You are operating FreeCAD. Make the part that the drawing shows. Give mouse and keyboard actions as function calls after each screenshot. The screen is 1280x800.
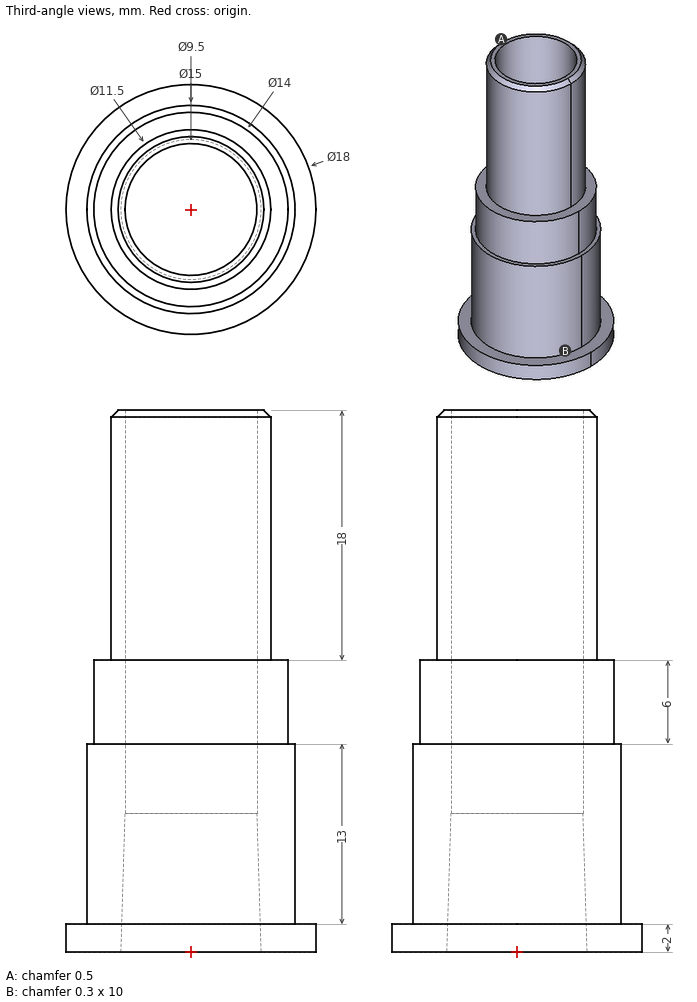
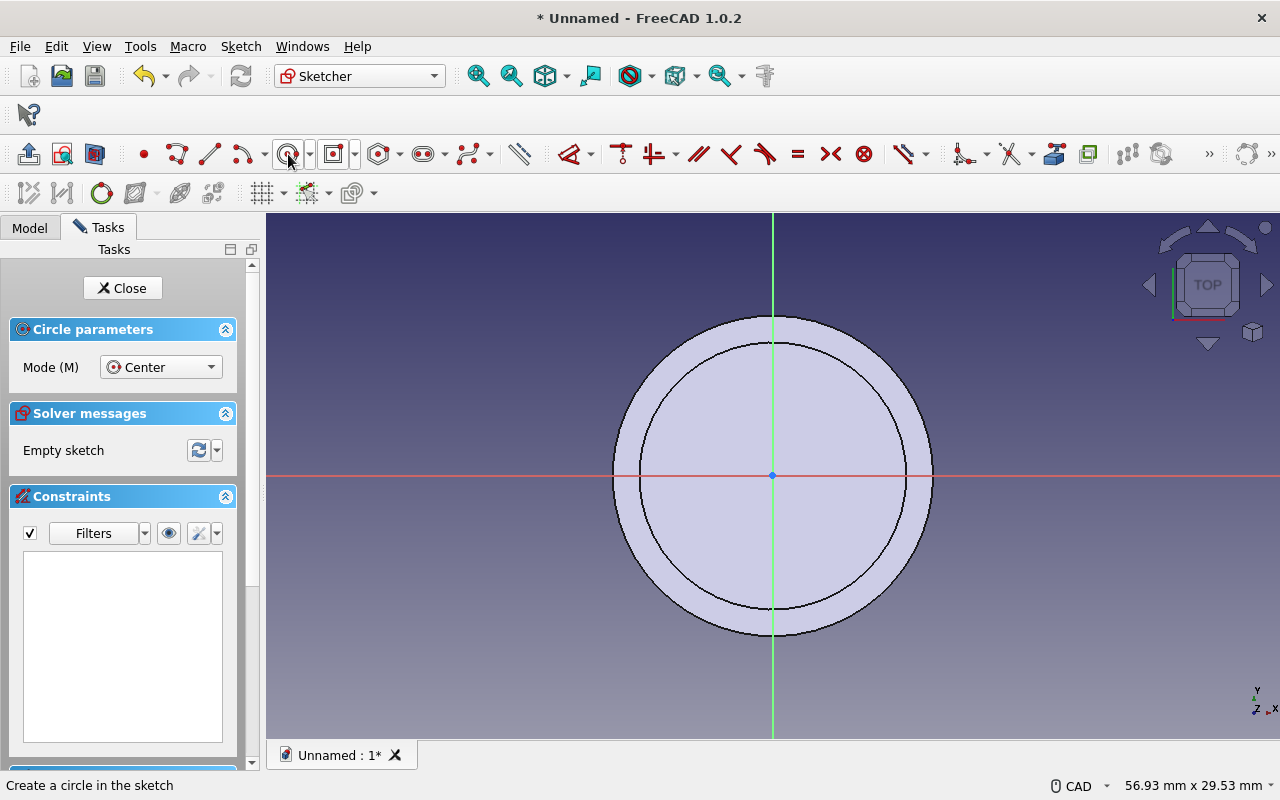
click(773, 476)
click(861, 388)
key(Escape)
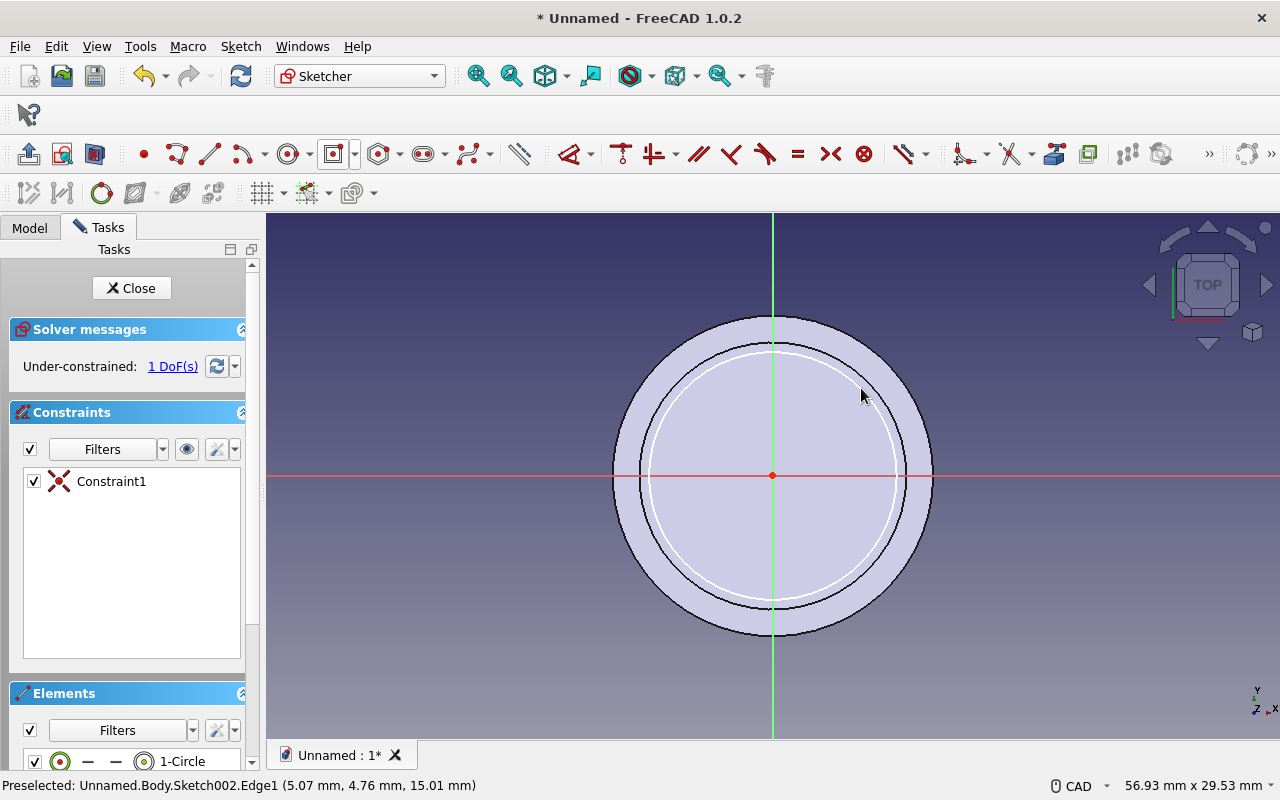
click(568, 154)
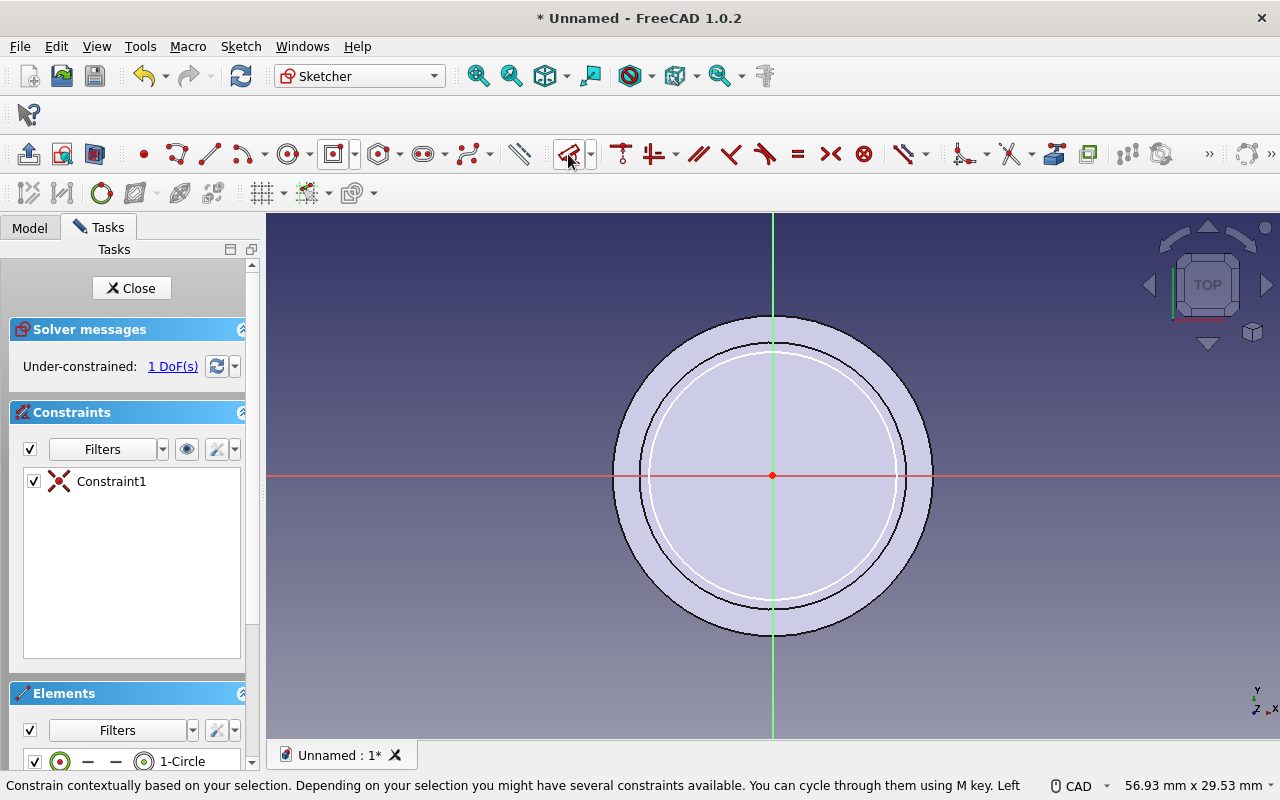
click(860, 388)
click(883, 365)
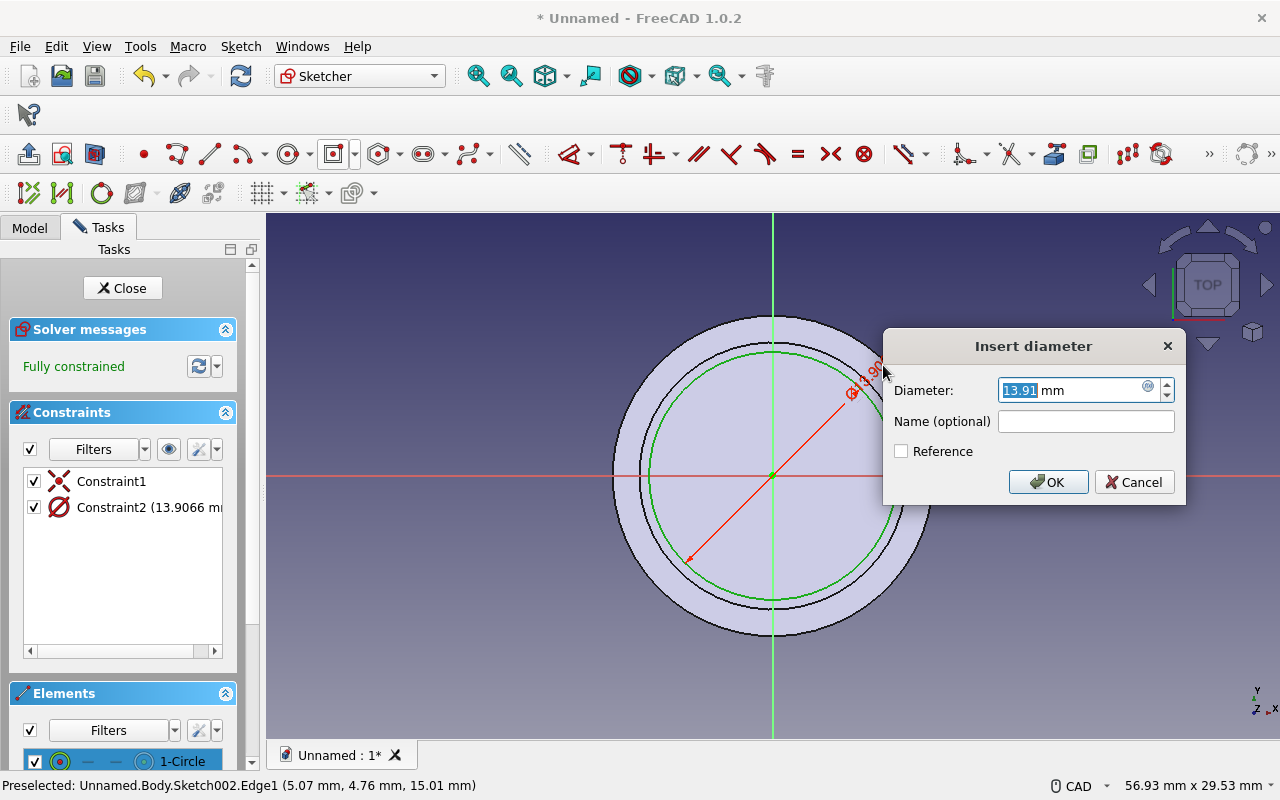
text(14)
key(Return)
key(Escape)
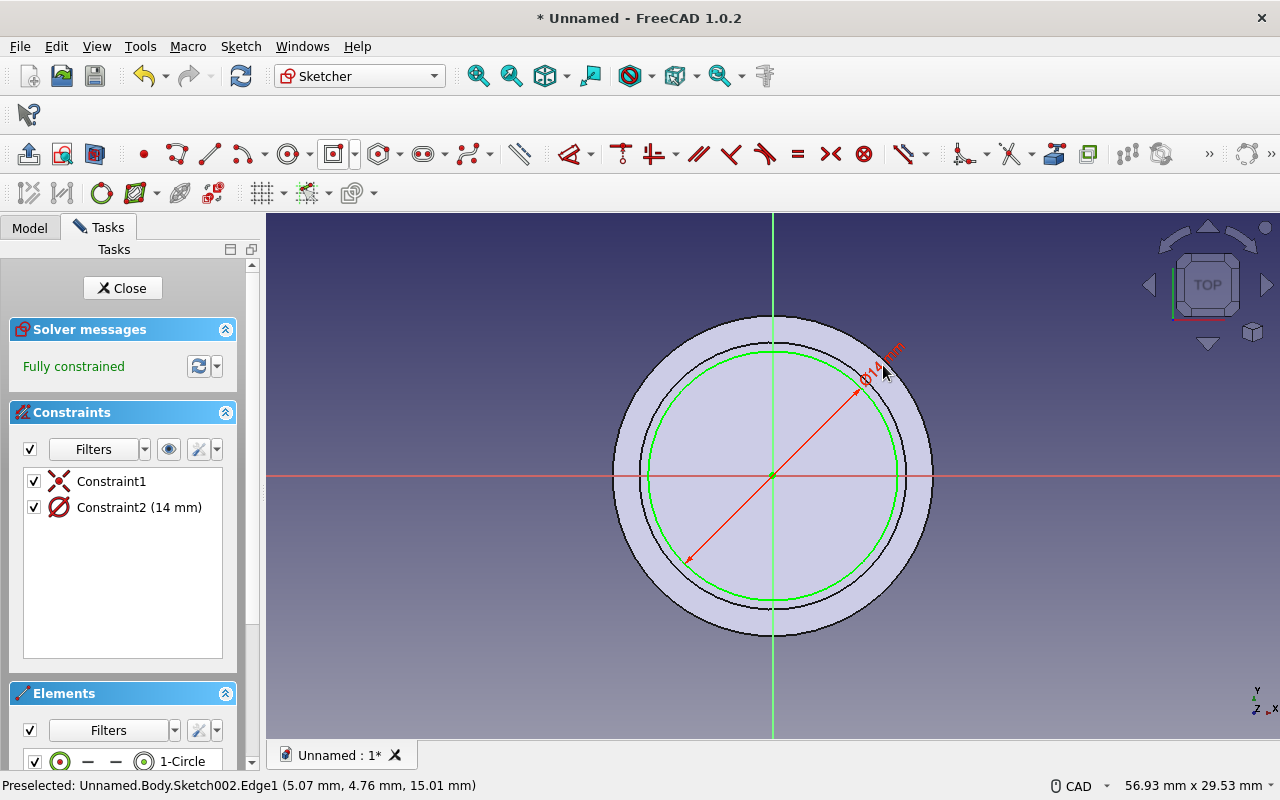
click(123, 288)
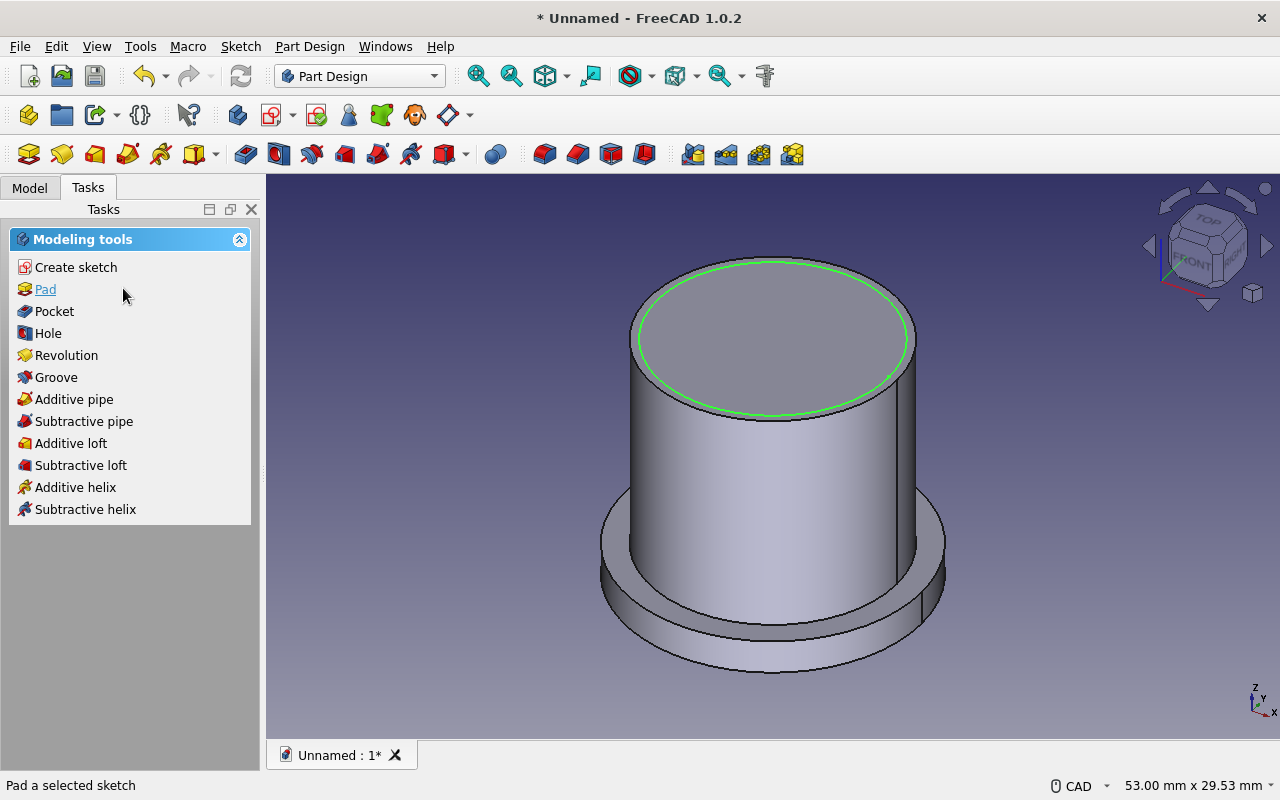
click(29, 154)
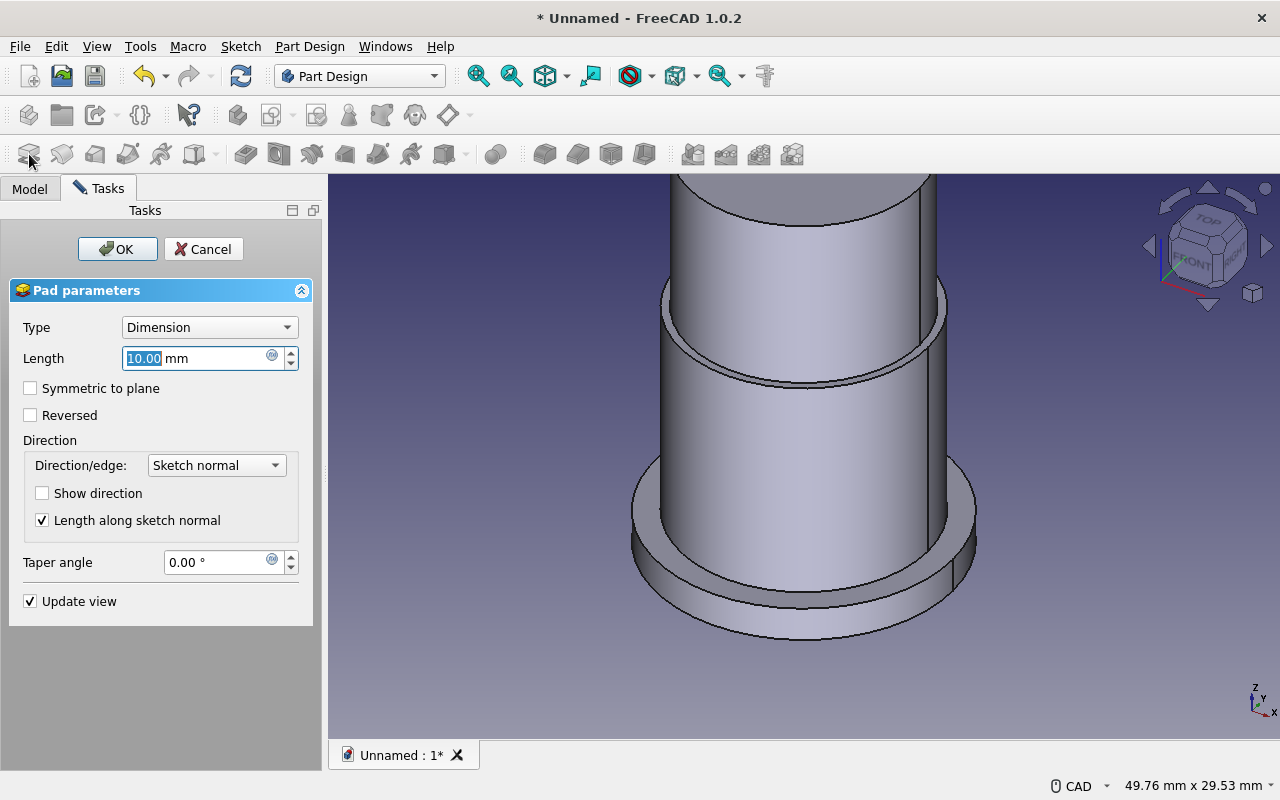
text(6)
key(Tab)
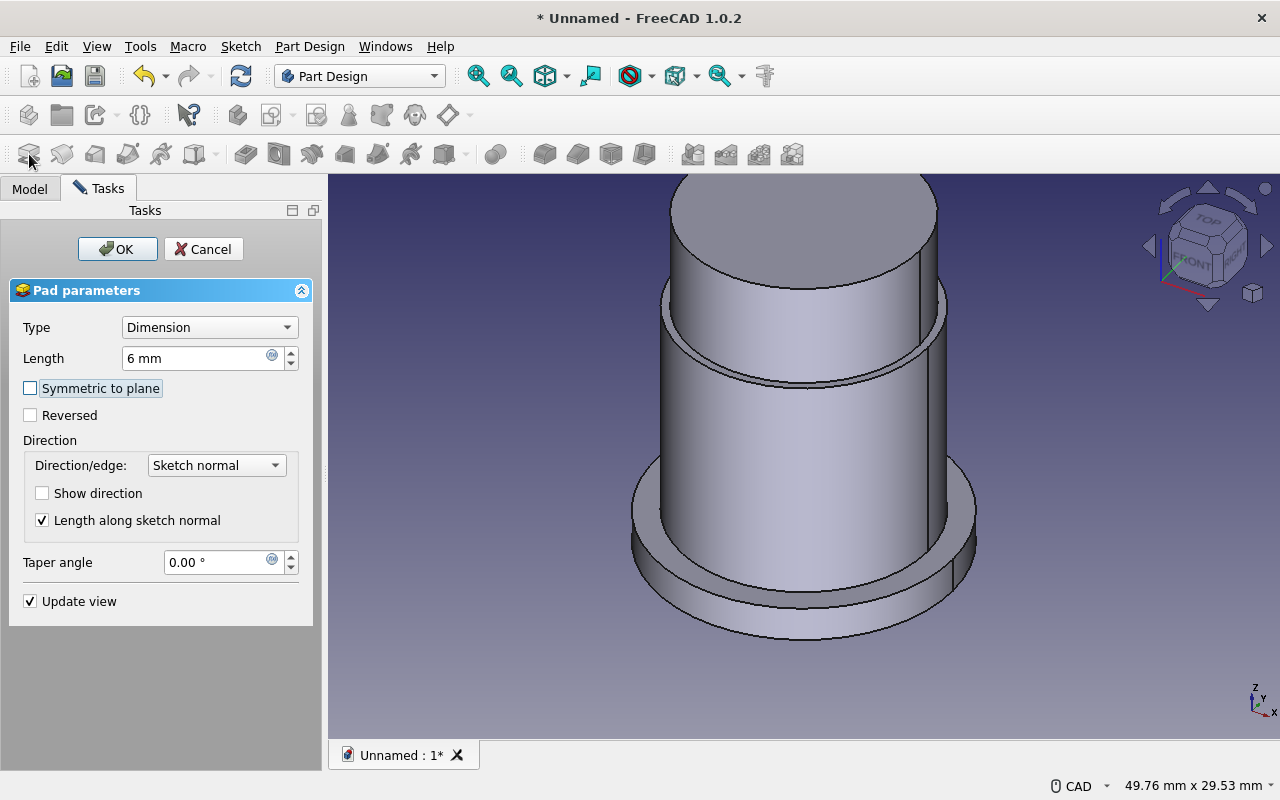
click(118, 249)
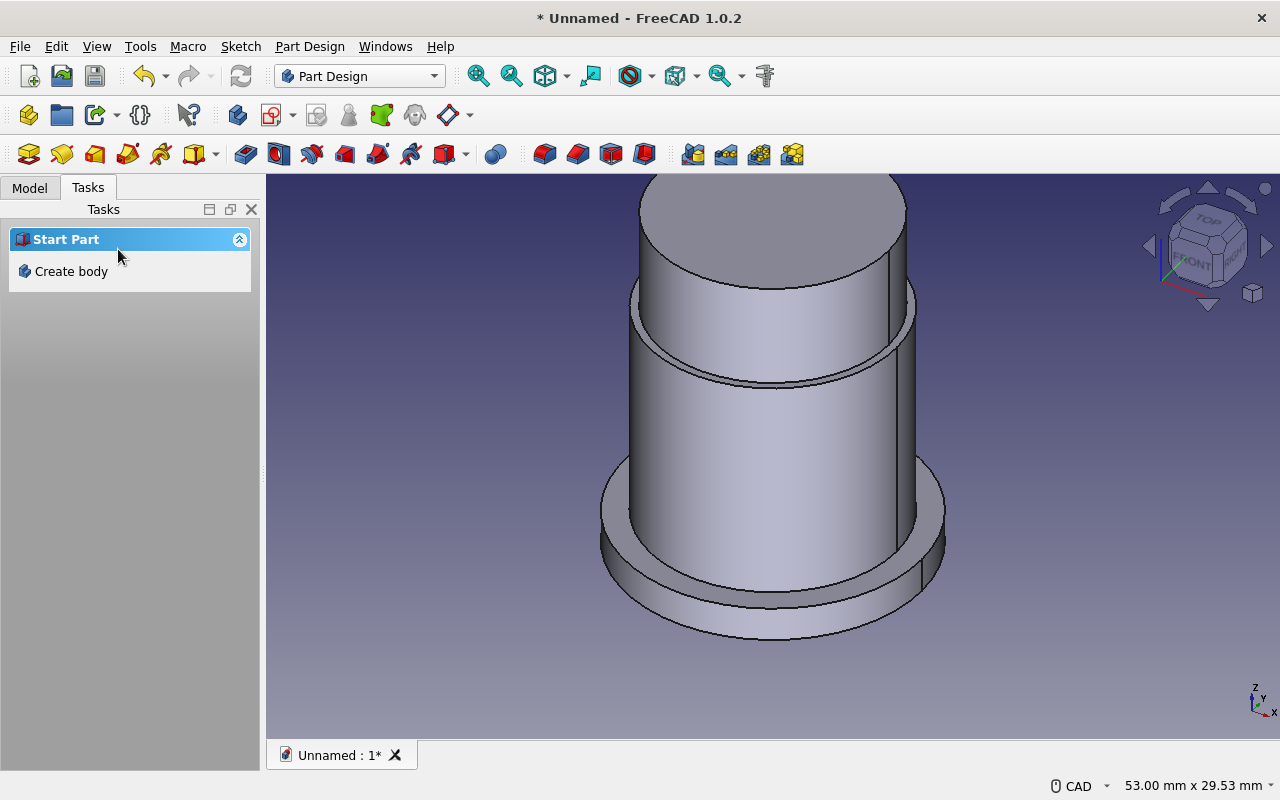
click(479, 76)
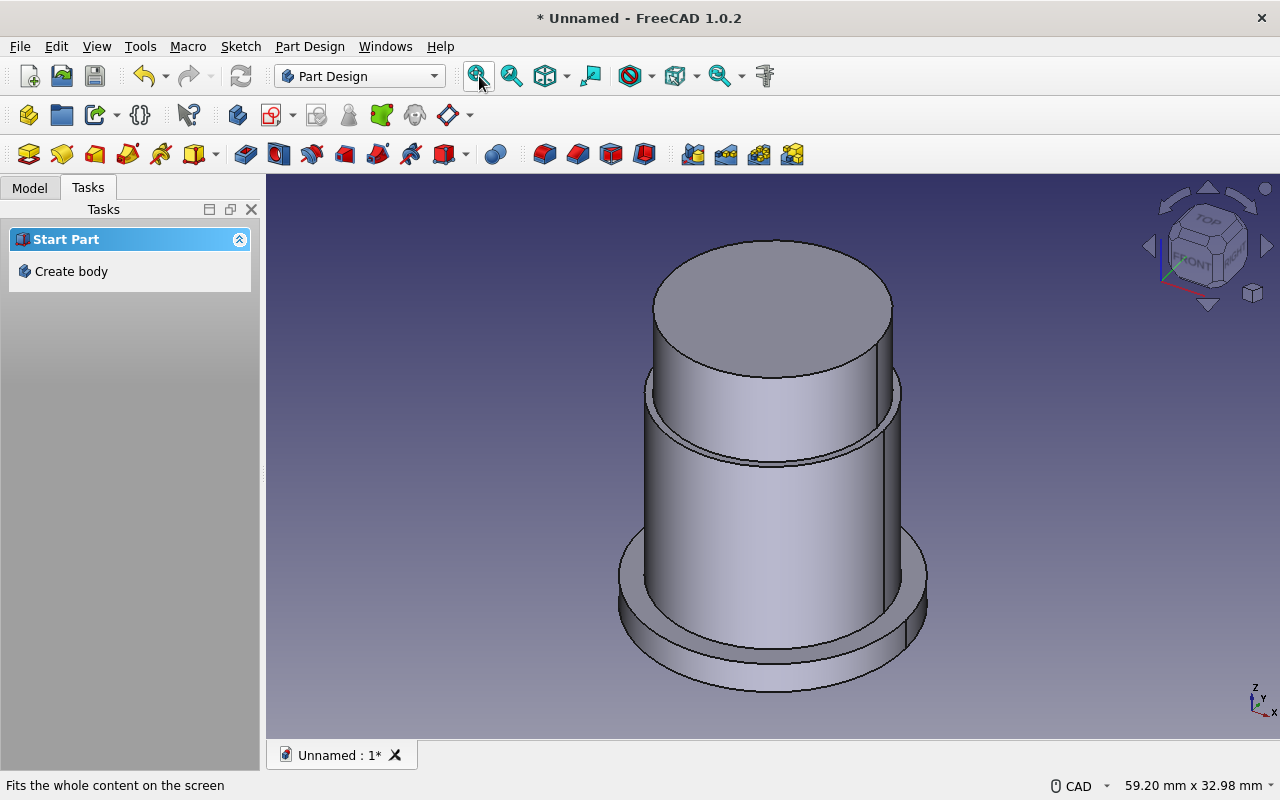
click(773, 308)